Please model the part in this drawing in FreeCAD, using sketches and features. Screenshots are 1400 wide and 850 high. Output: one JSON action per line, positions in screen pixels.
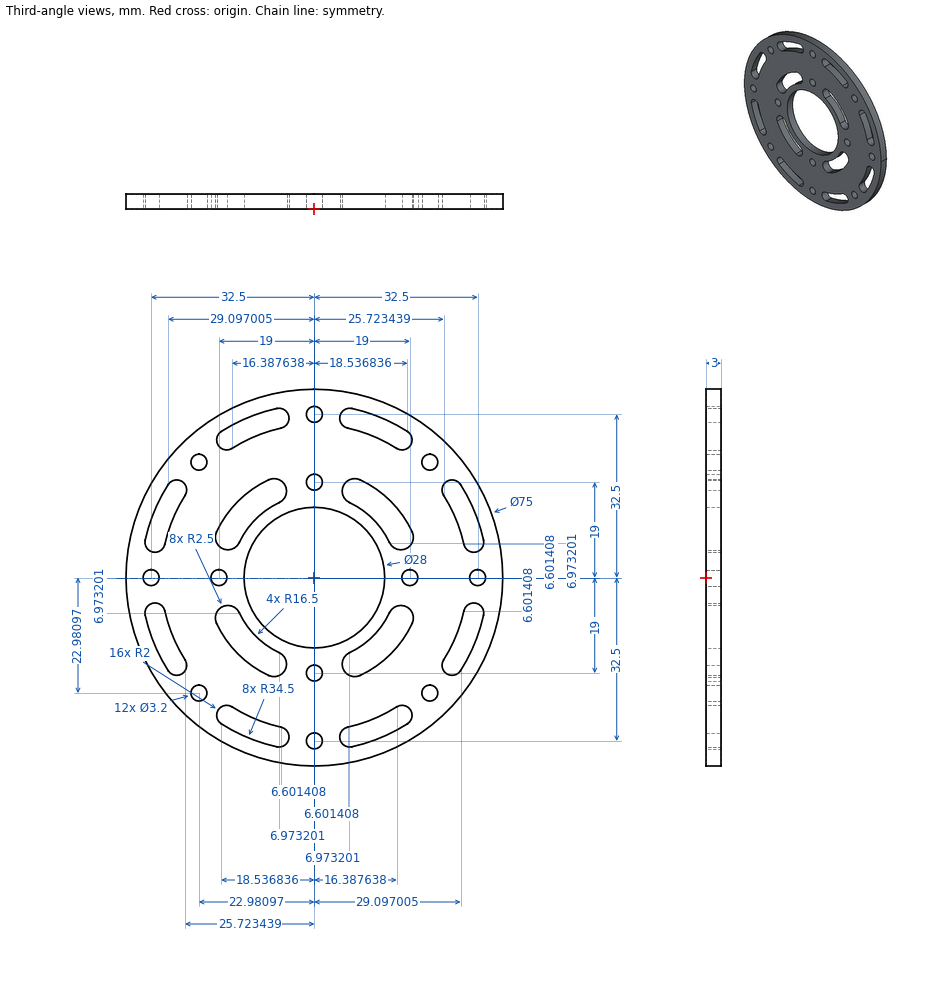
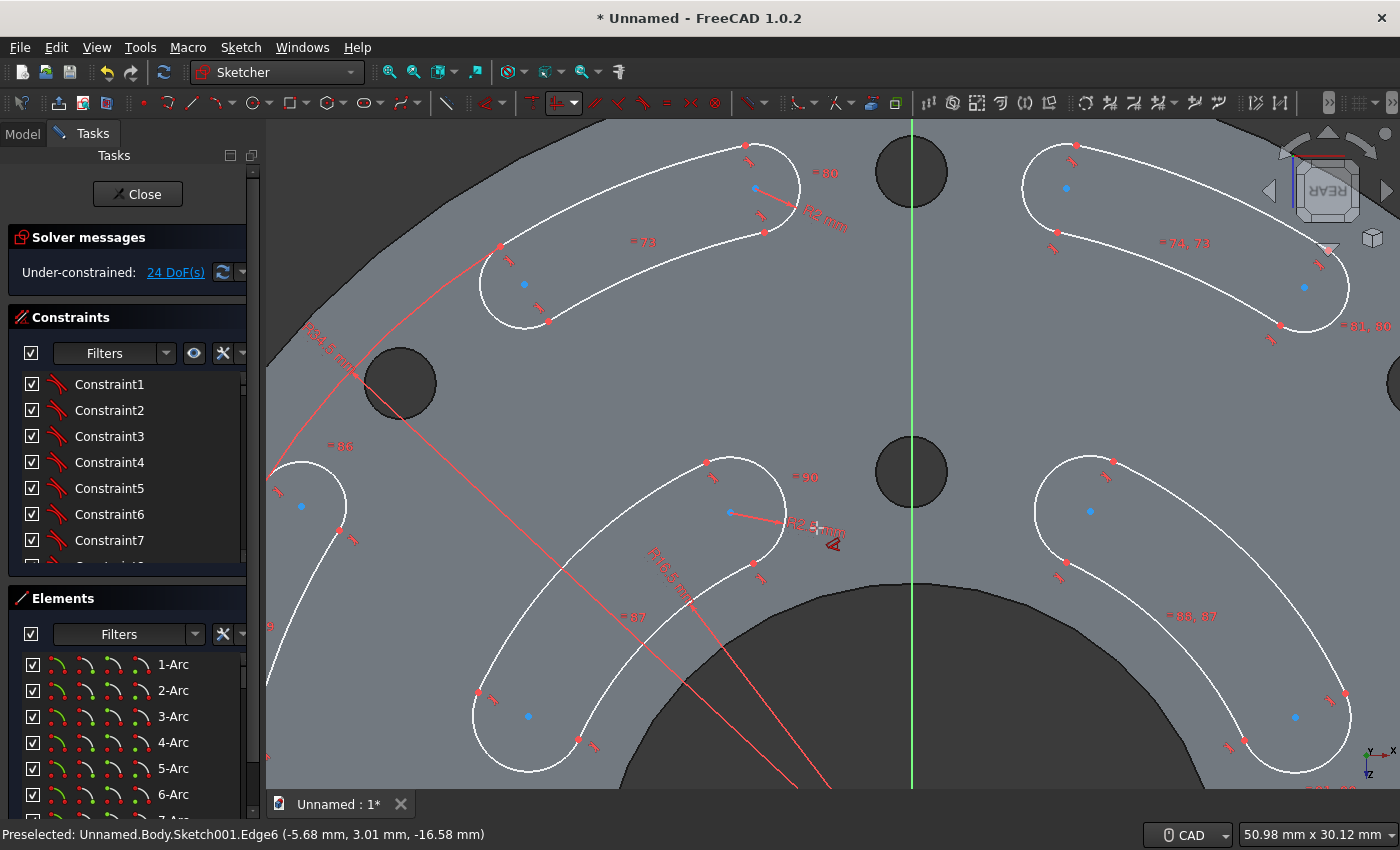
{"action": "left_click", "coordinate": [765, 232]}
{"action": "left_click", "coordinate": [838, 174]}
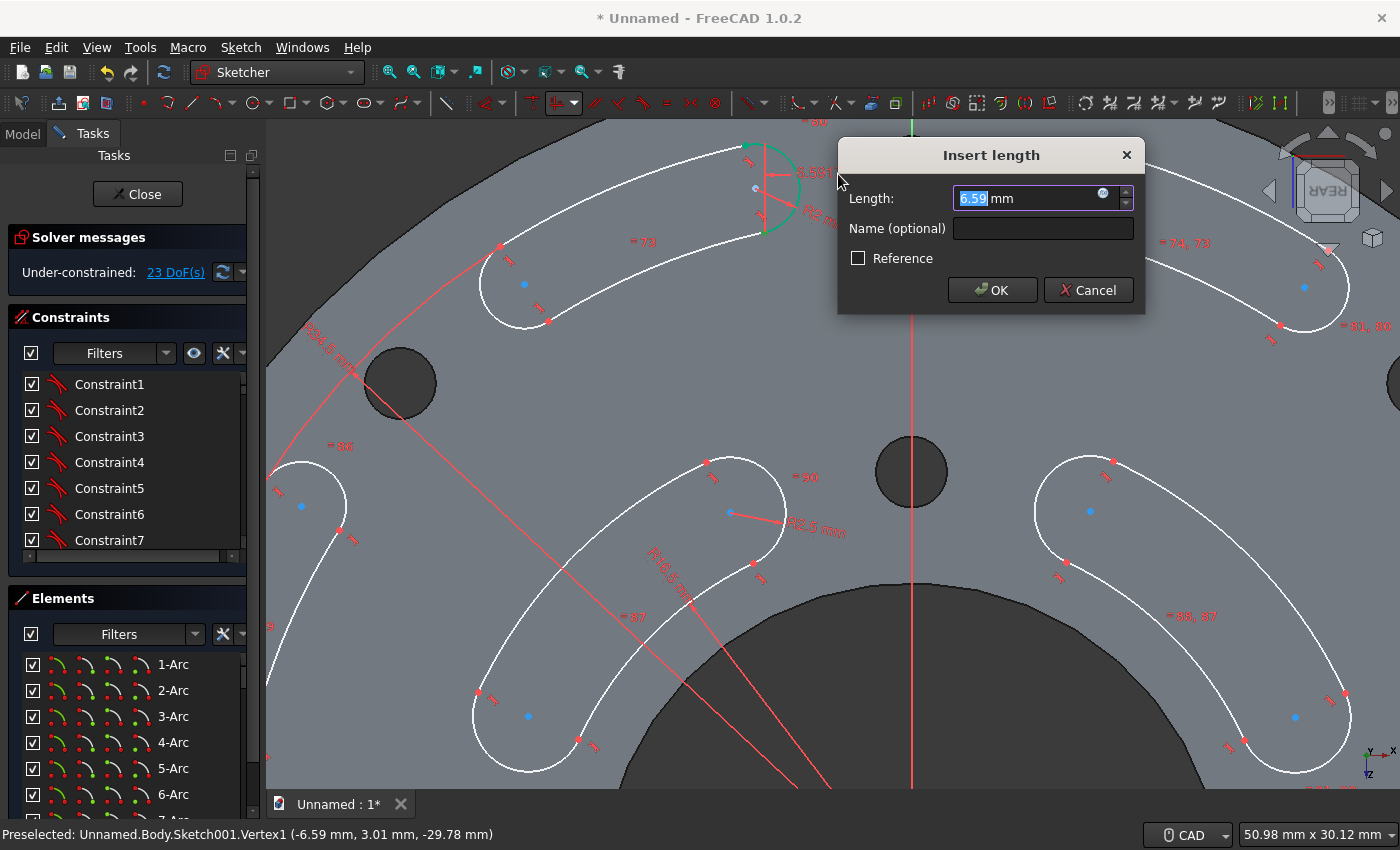
{"action": "type", "text": "6.601408"}
{"action": "key", "text": "Return"}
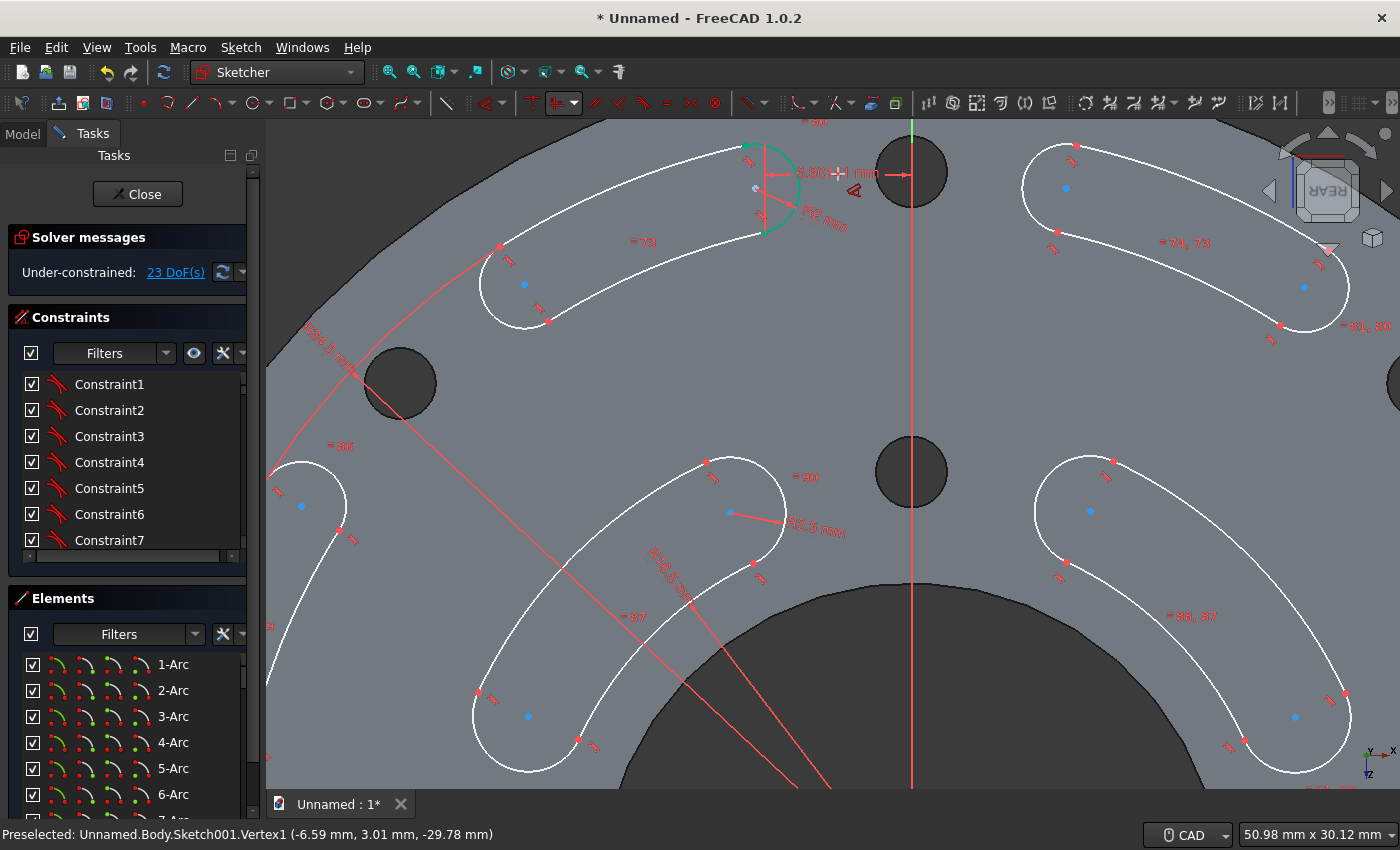
{"action": "left_click", "coordinate": [754, 563]}
{"action": "left_click", "coordinate": [888, 529]}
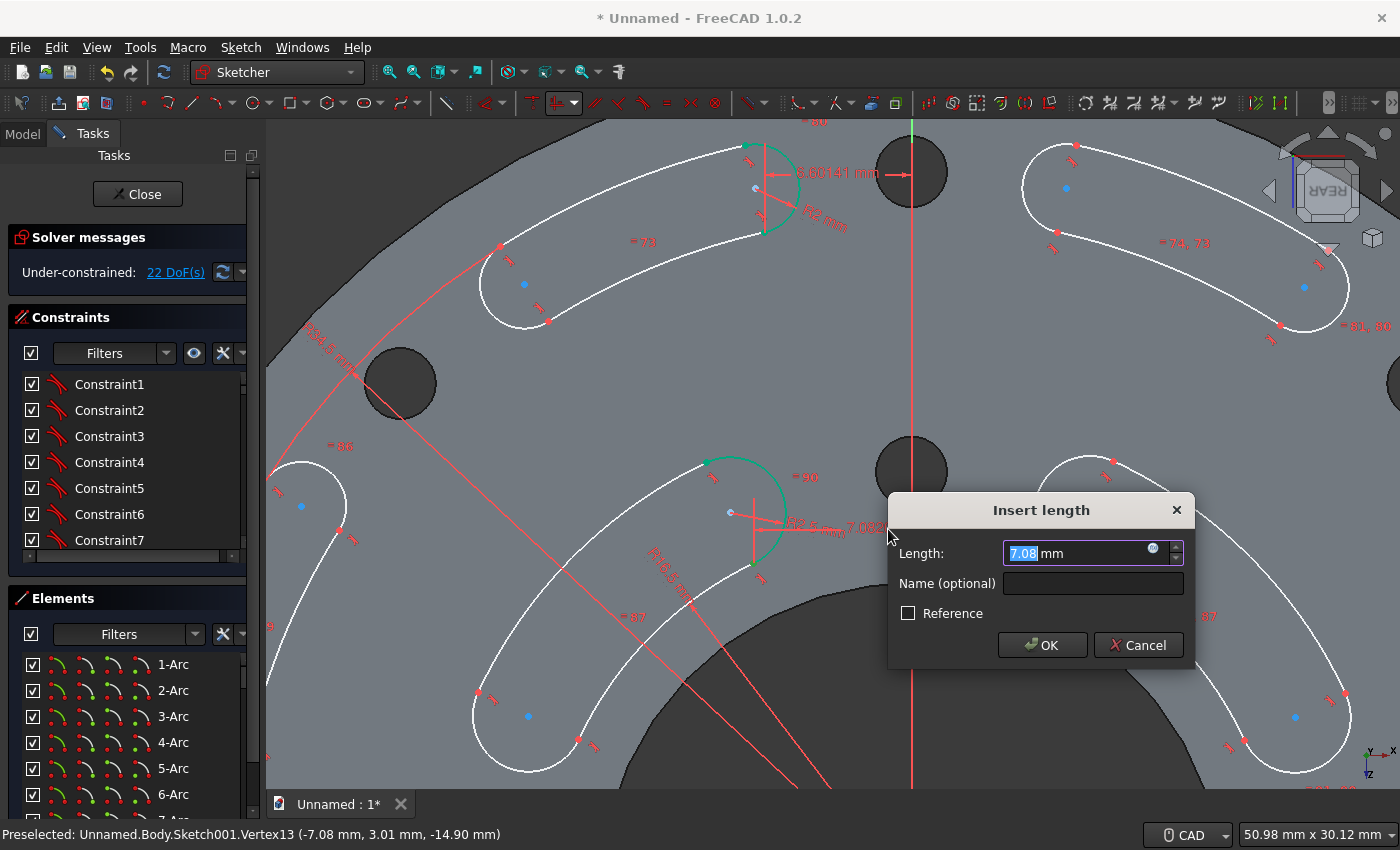
{"action": "type", "text": "6.973201"}
{"action": "key", "text": "Return"}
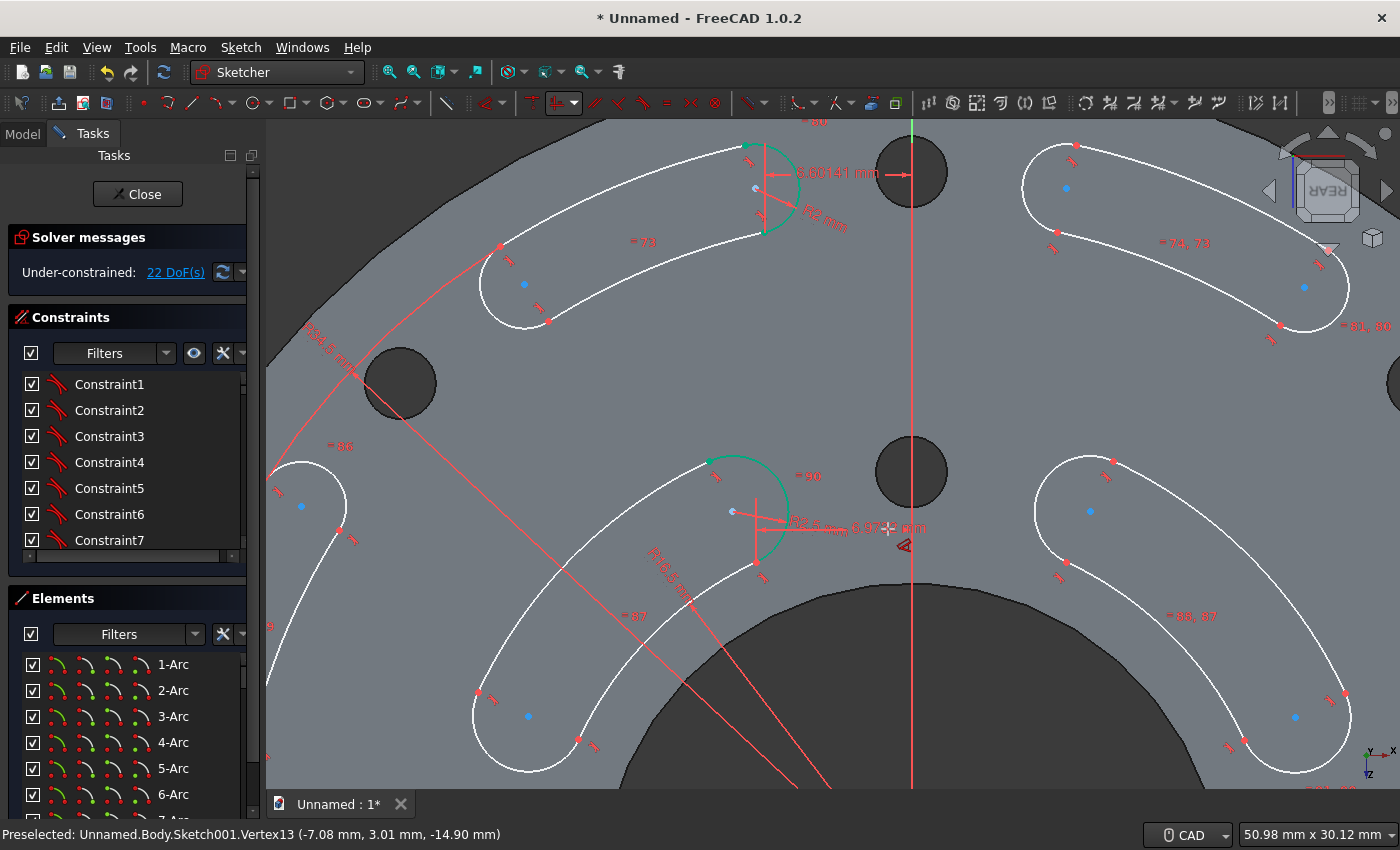
{"action": "left_click", "coordinate": [579, 740]}
{"action": "left_click", "coordinate": [545, 750]}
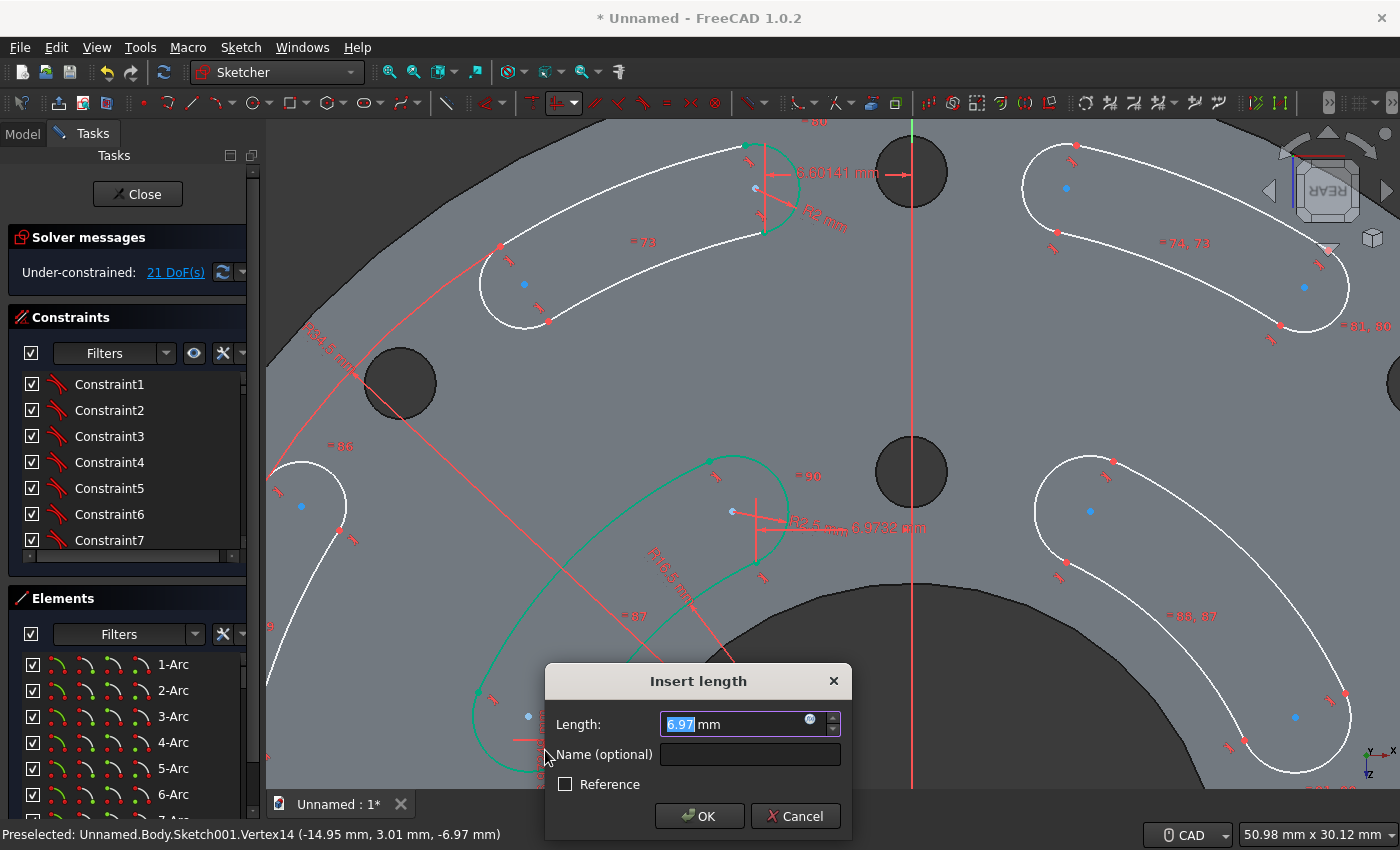
{"action": "type", "text": "6.973201"}
{"action": "key", "text": "Return"}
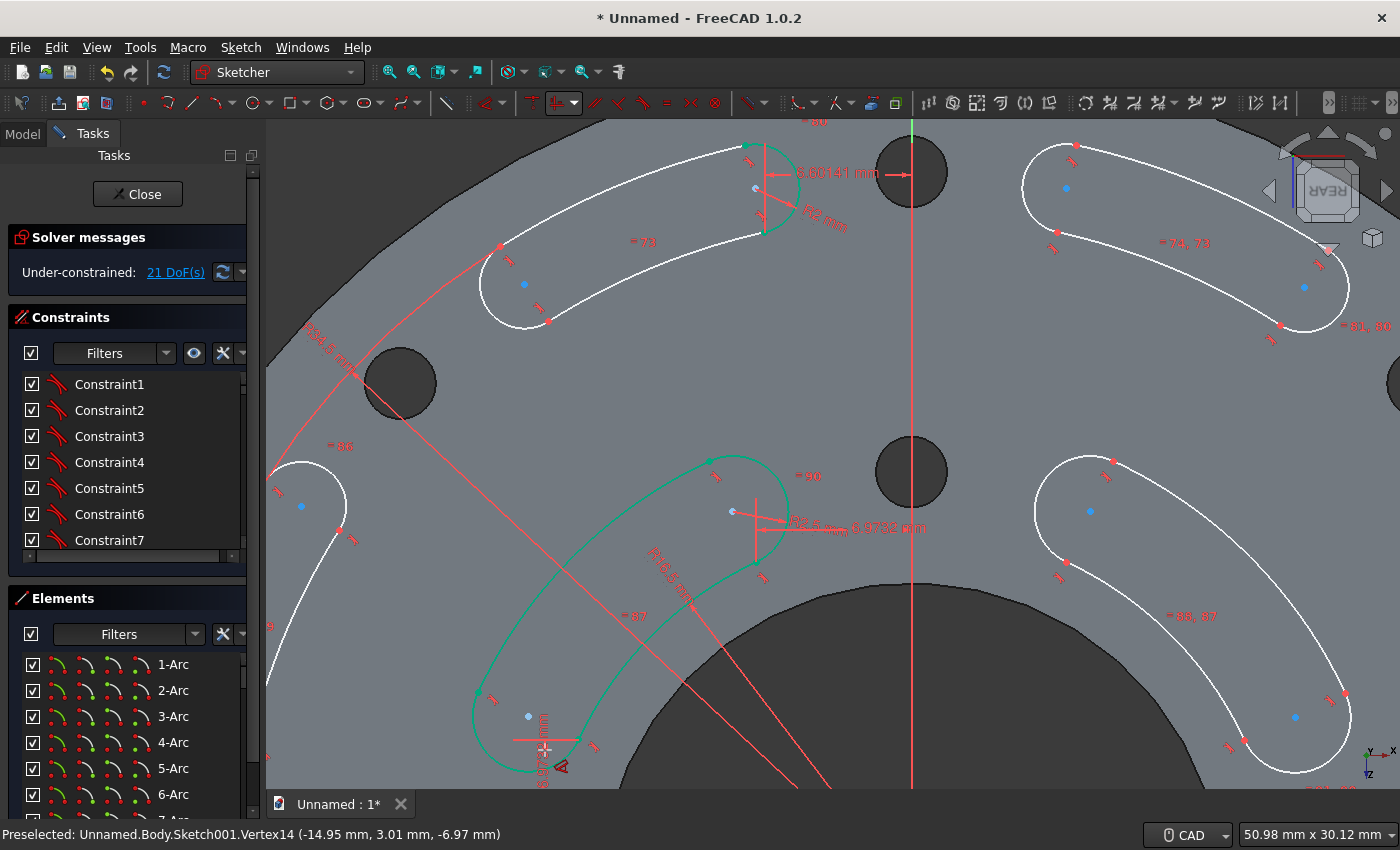
{"action": "left_click", "coordinate": [1057, 232]}
{"action": "left_click", "coordinate": [984, 198]}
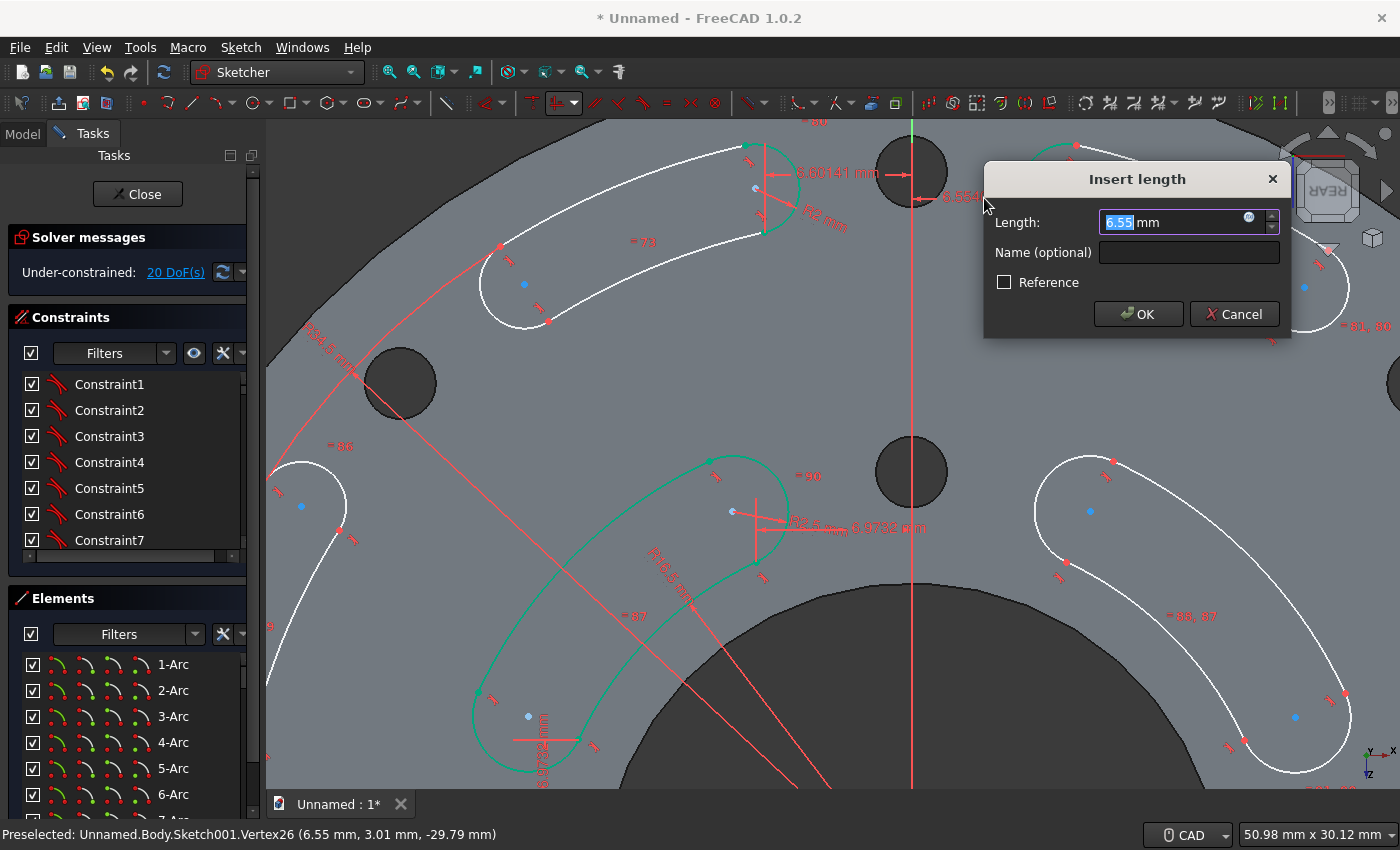
{"action": "type", "text": "6.601408"}
{"action": "key", "text": "Return"}